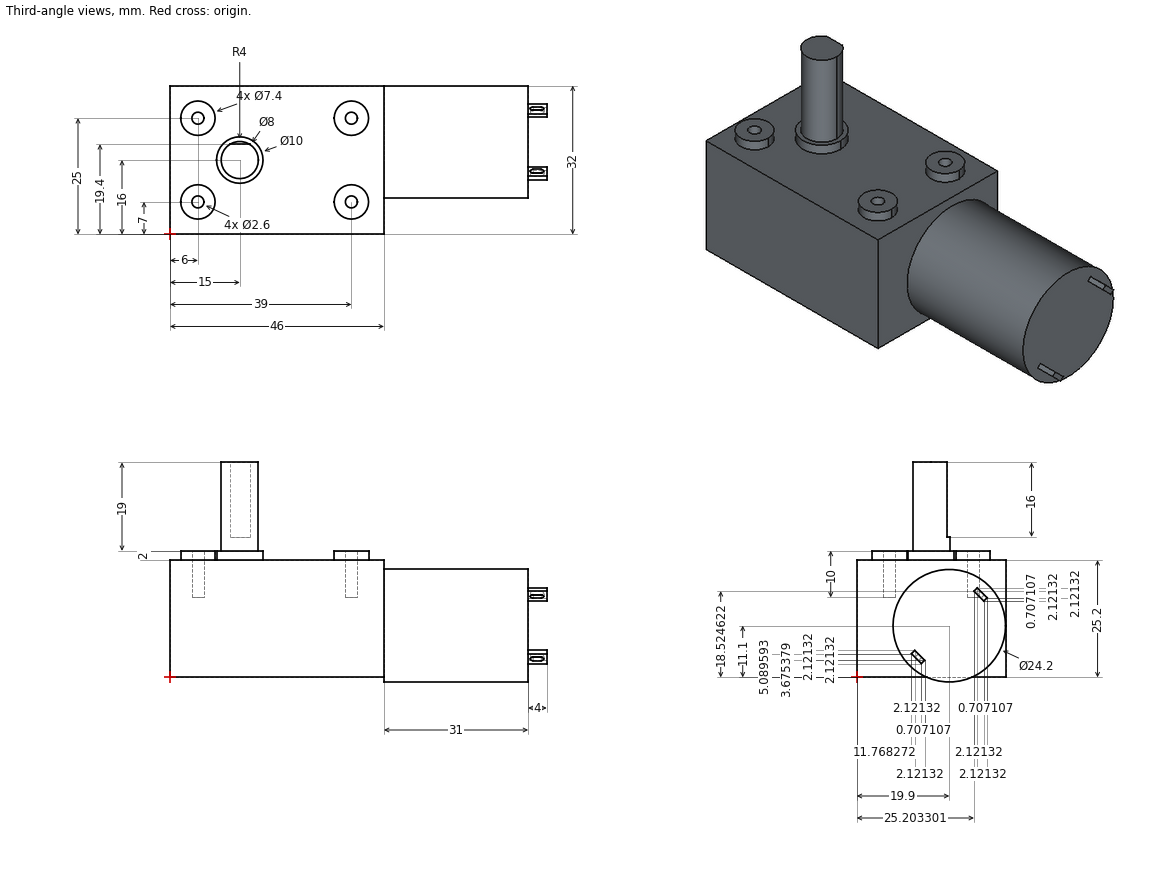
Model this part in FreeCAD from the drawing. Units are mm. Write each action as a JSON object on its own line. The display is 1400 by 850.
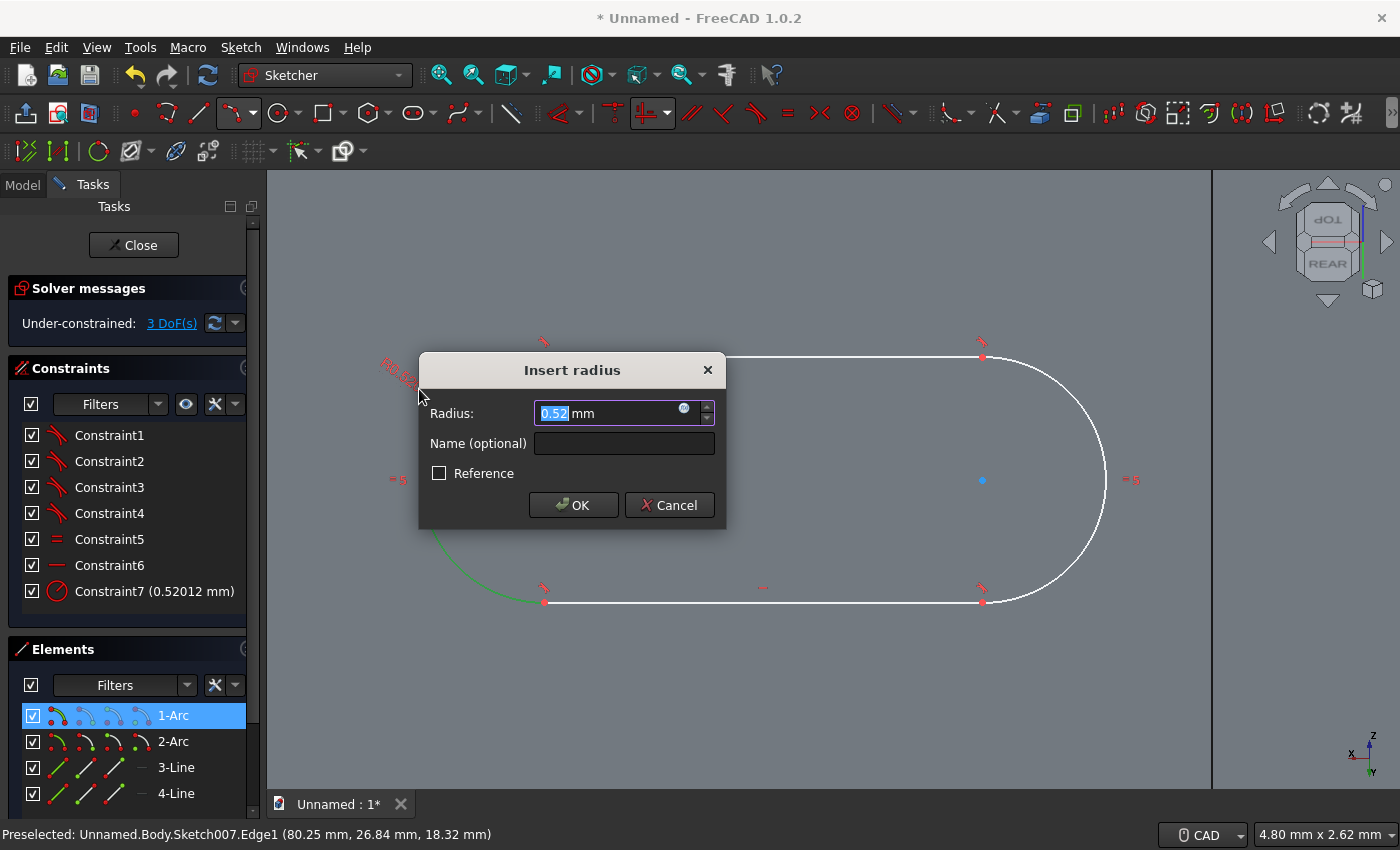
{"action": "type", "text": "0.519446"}
{"action": "key", "text": "Return"}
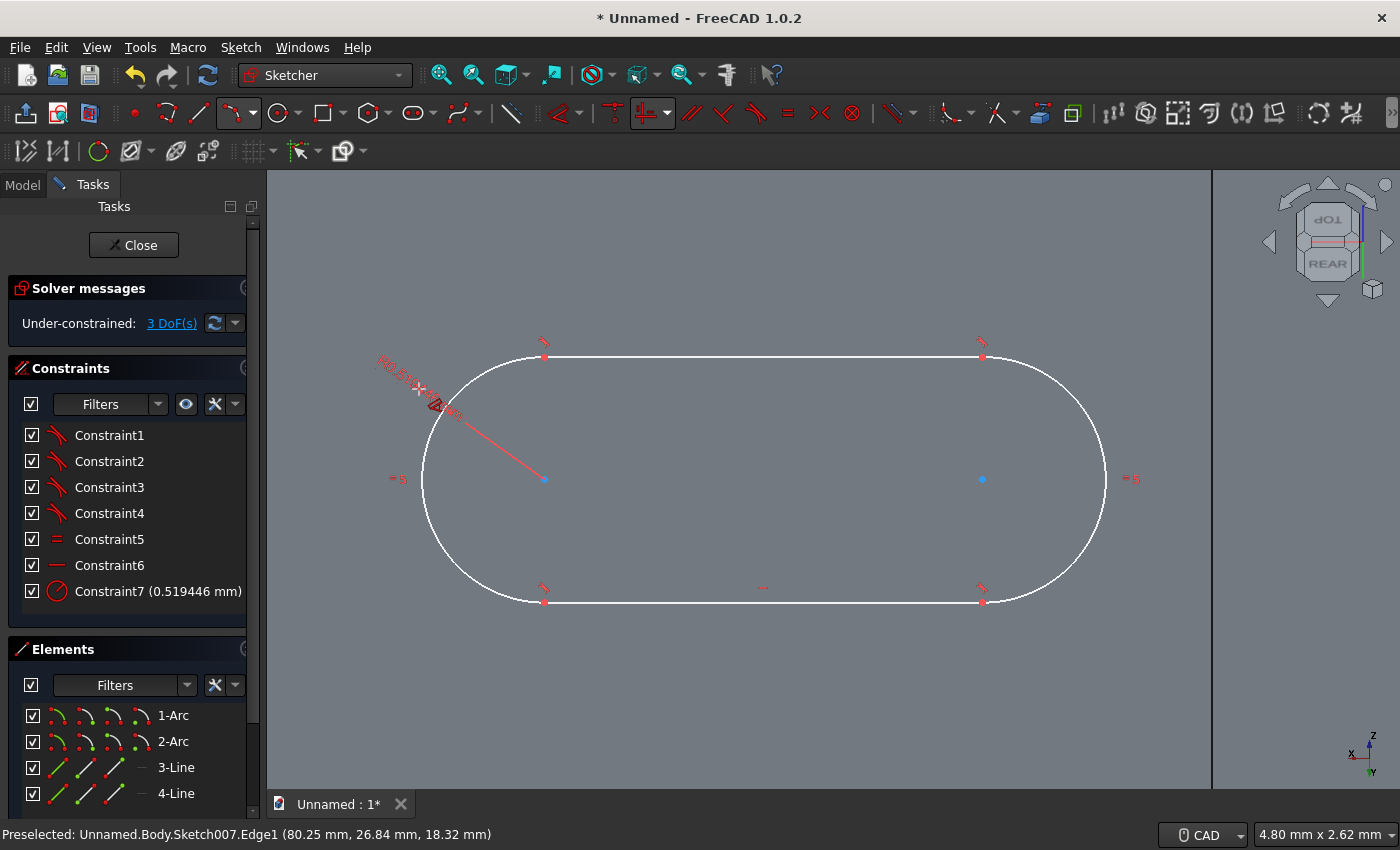
{"action": "left_click", "coordinate": [676, 357]}
{"action": "left_click", "coordinate": [764, 323]}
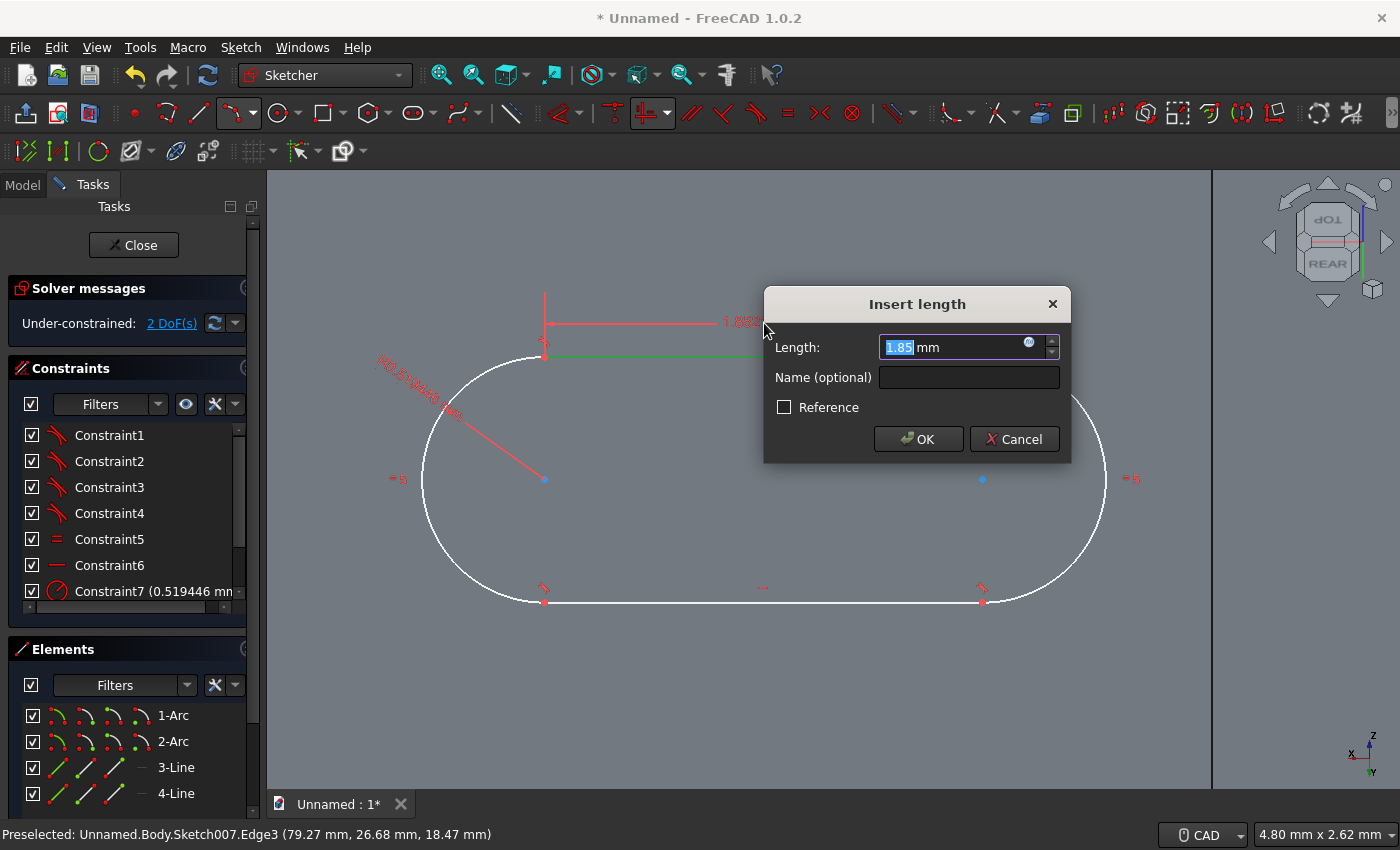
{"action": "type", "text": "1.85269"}
{"action": "key", "text": "Return"}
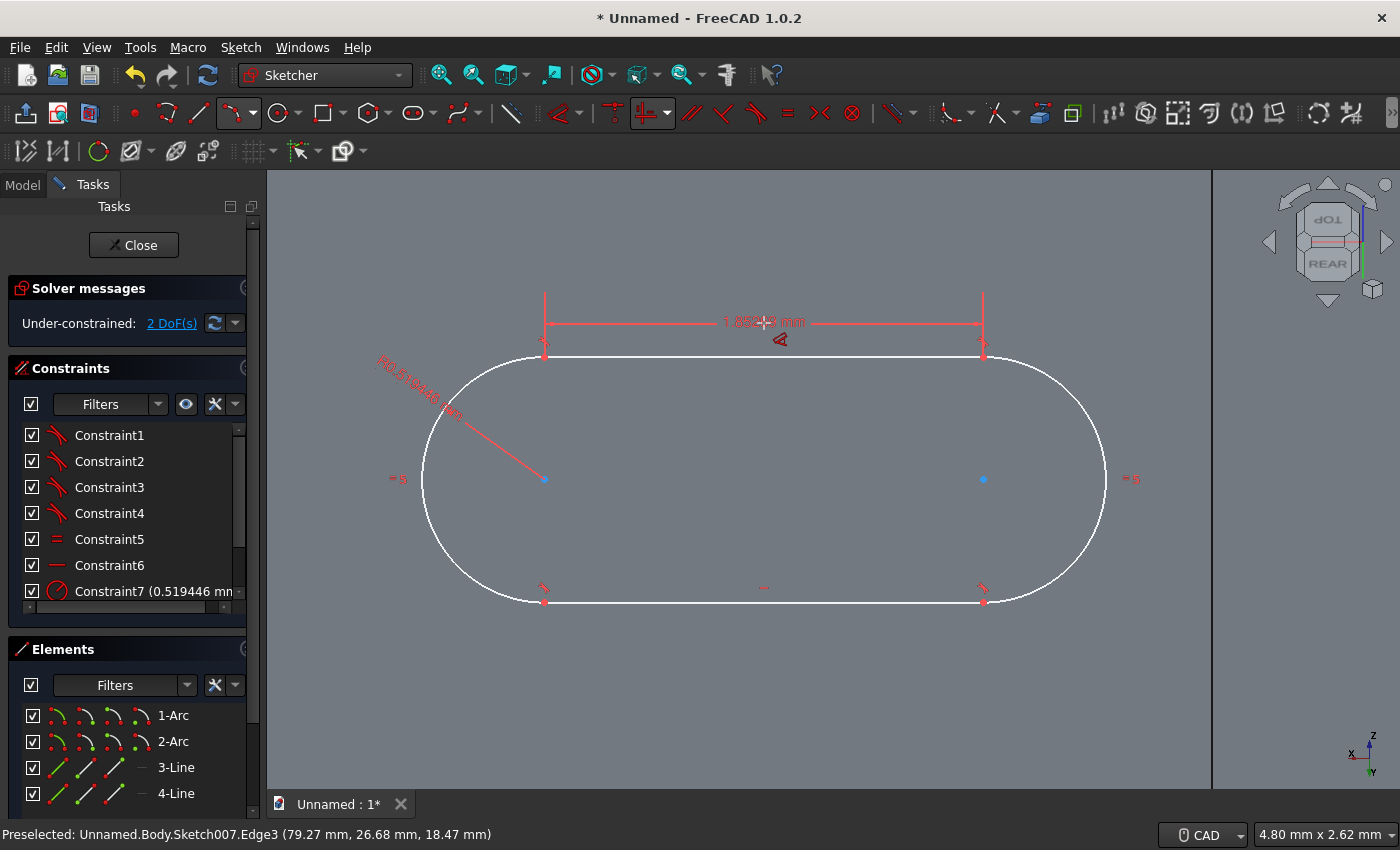
{"action": "left_click", "coordinate": [545, 357]}
{"action": "left_click", "coordinate": [511, 278]}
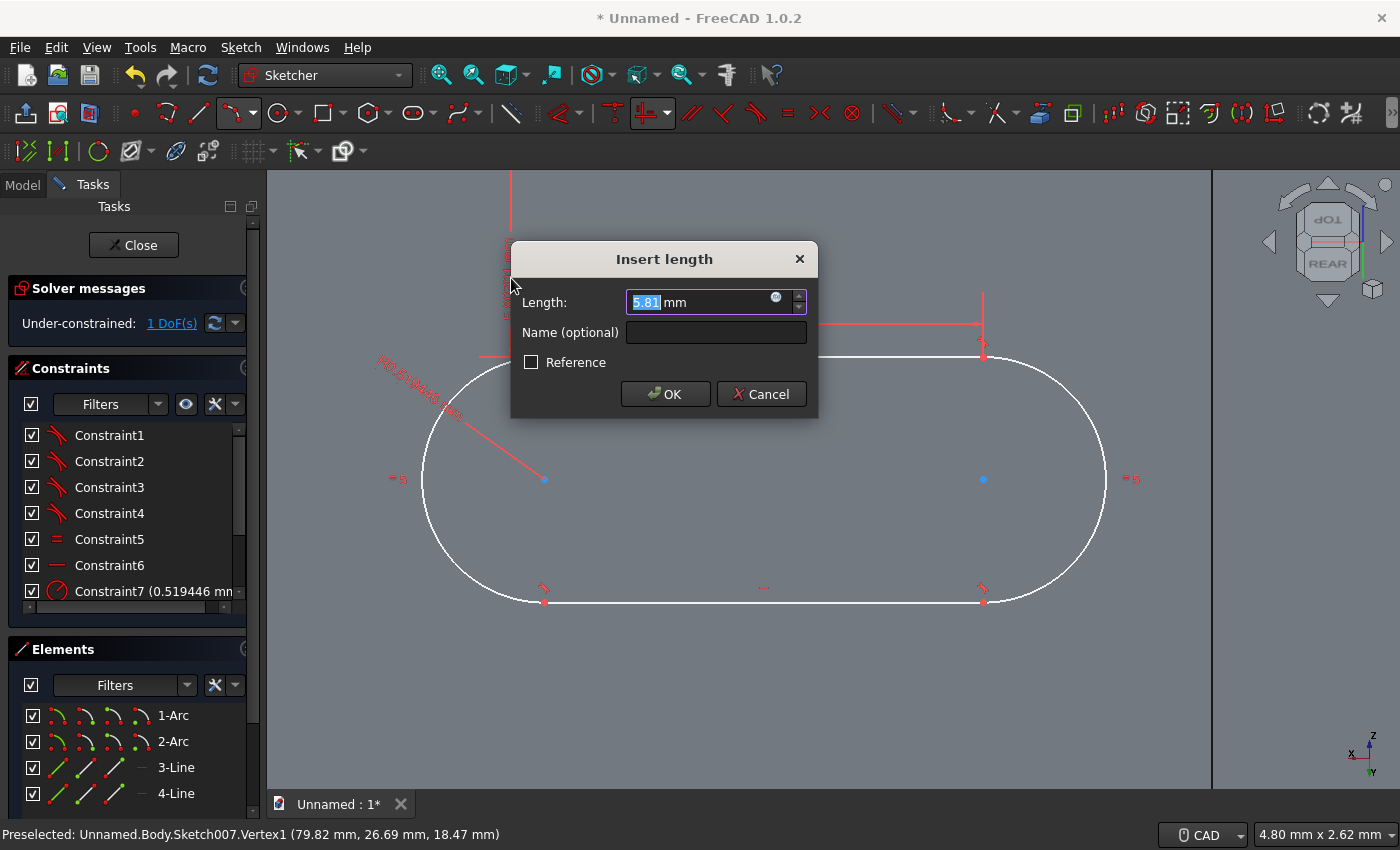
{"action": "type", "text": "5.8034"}
{"action": "key", "text": "Return"}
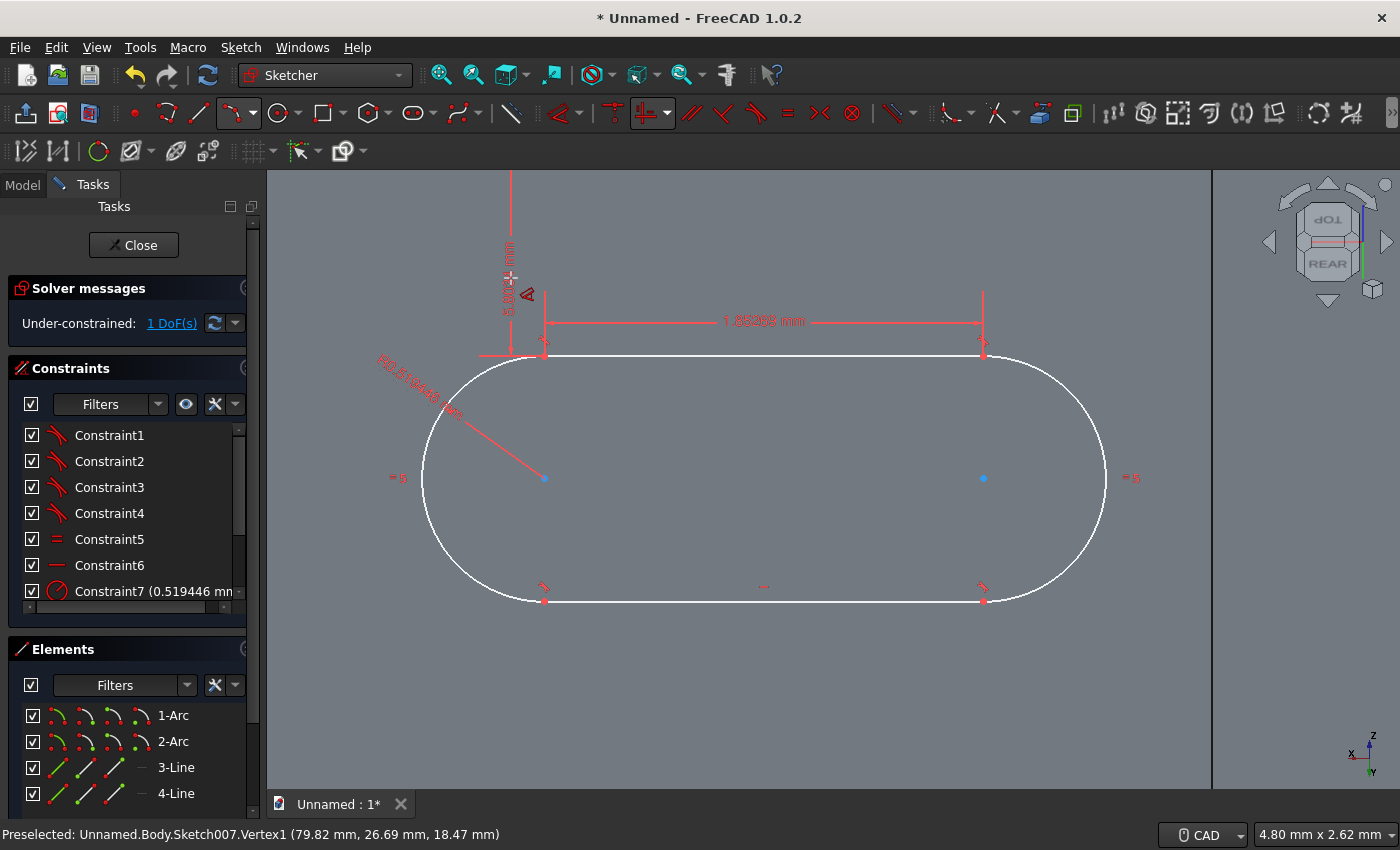
{"action": "left_click", "coordinate": [545, 356]}
{"action": "left_click", "coordinate": [890, 390]}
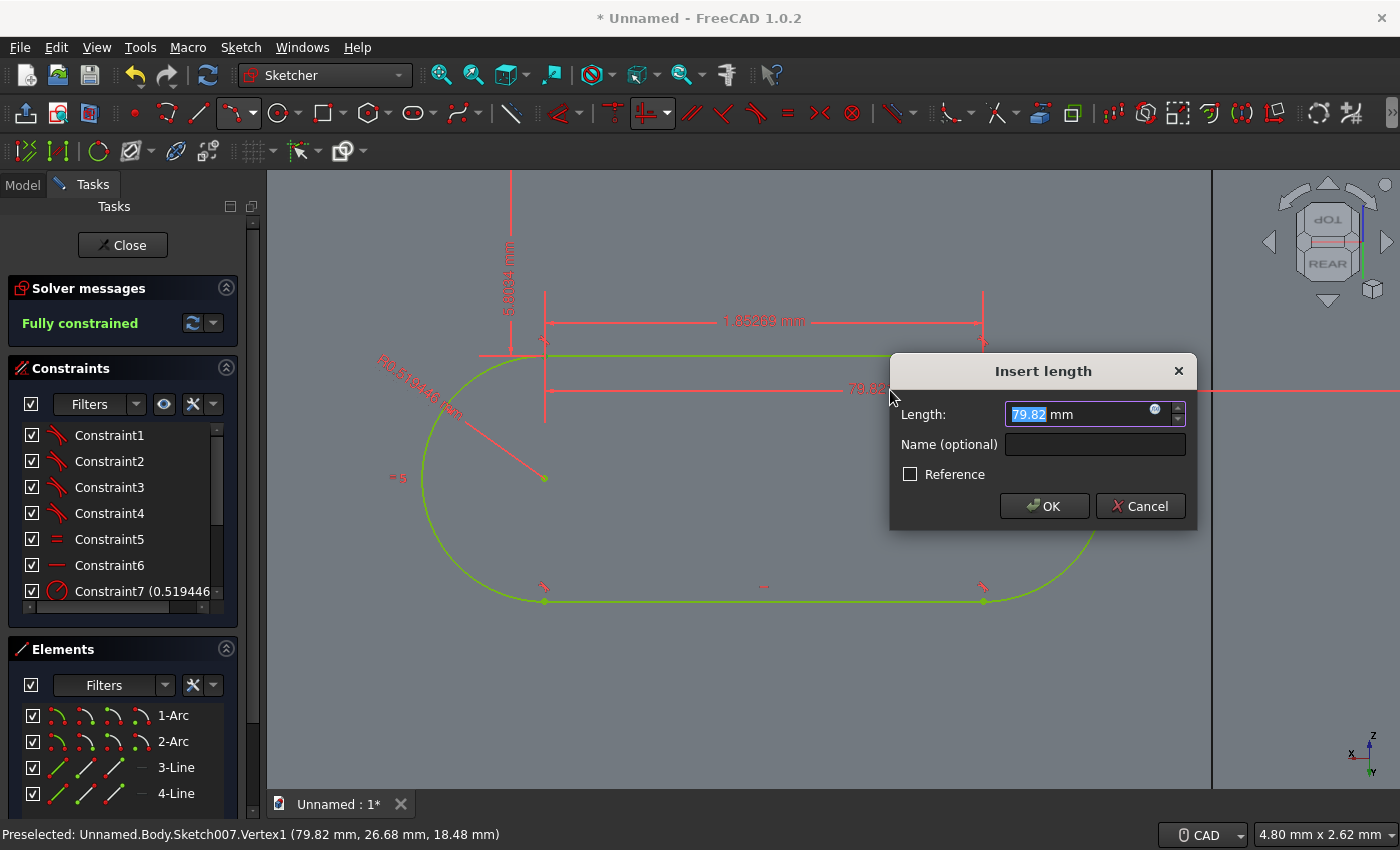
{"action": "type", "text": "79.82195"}
{"action": "key", "text": "Return"}
{"action": "key", "text": "Escape"}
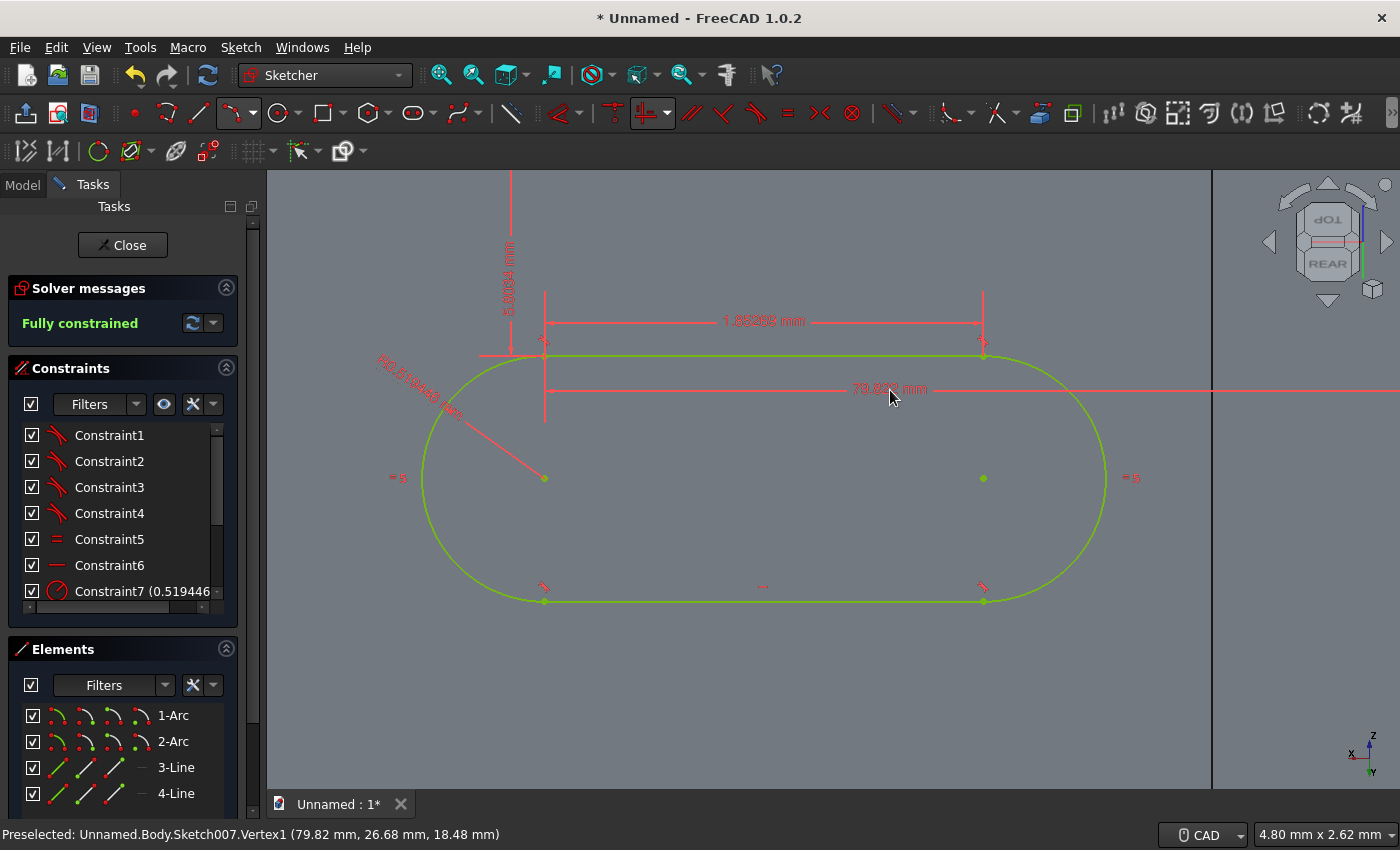
{"action": "left_click", "coordinate": [123, 245]}